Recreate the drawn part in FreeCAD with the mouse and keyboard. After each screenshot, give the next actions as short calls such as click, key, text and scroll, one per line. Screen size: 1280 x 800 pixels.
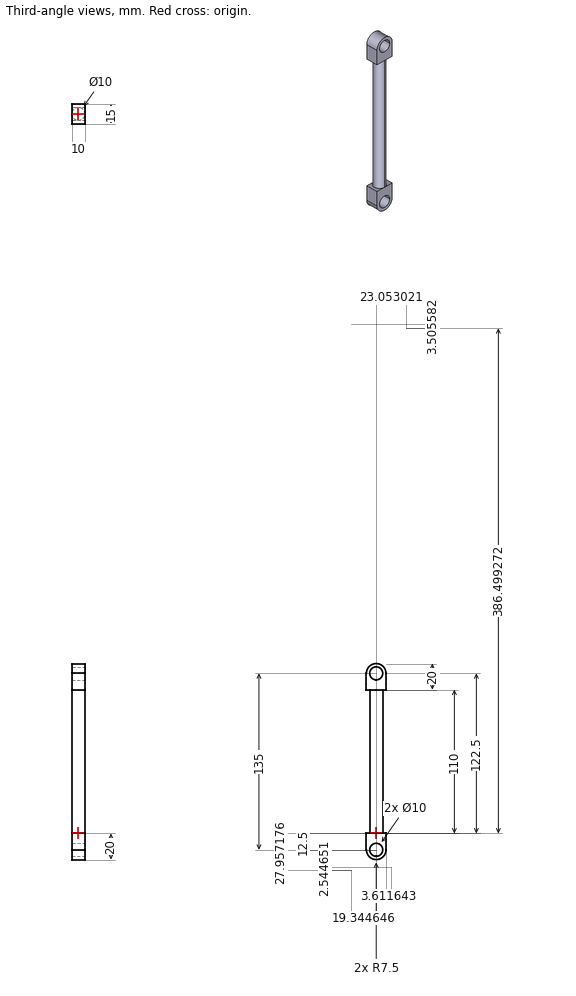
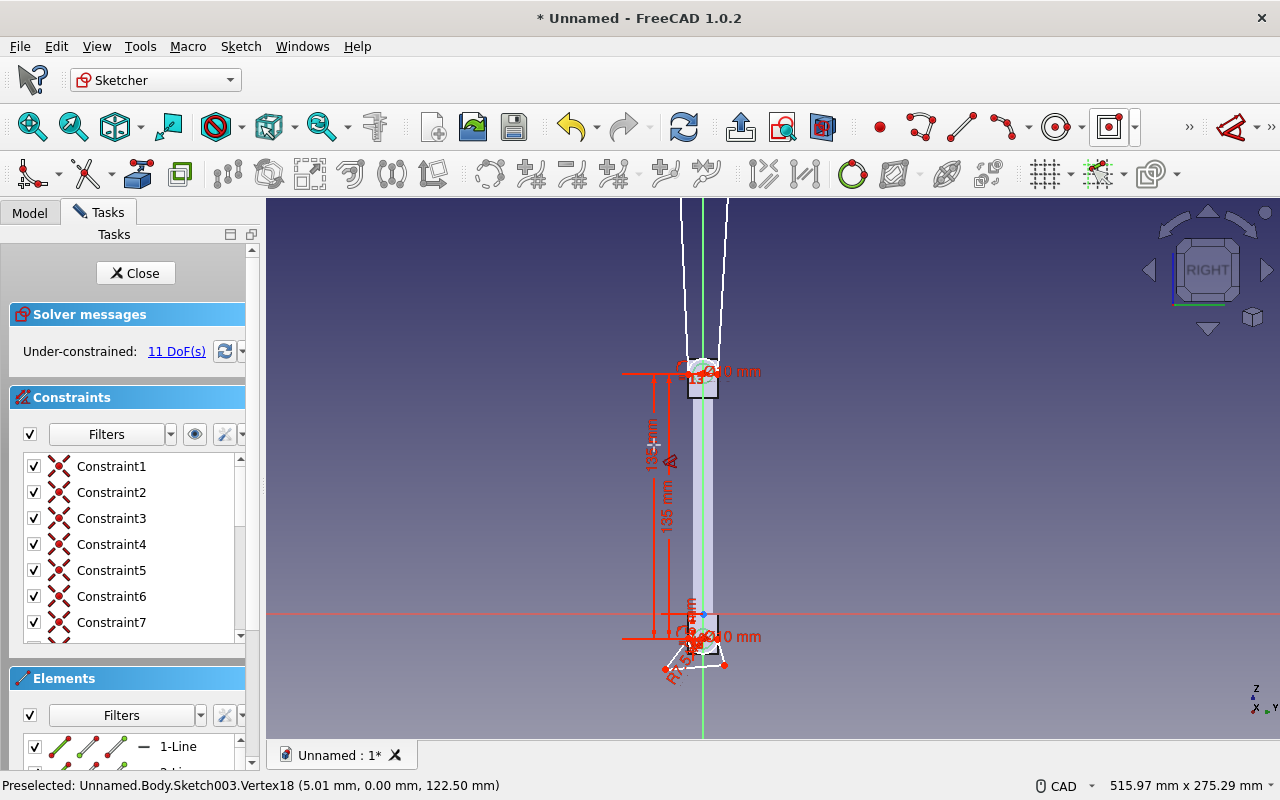
scroll(718, 640, up, 3)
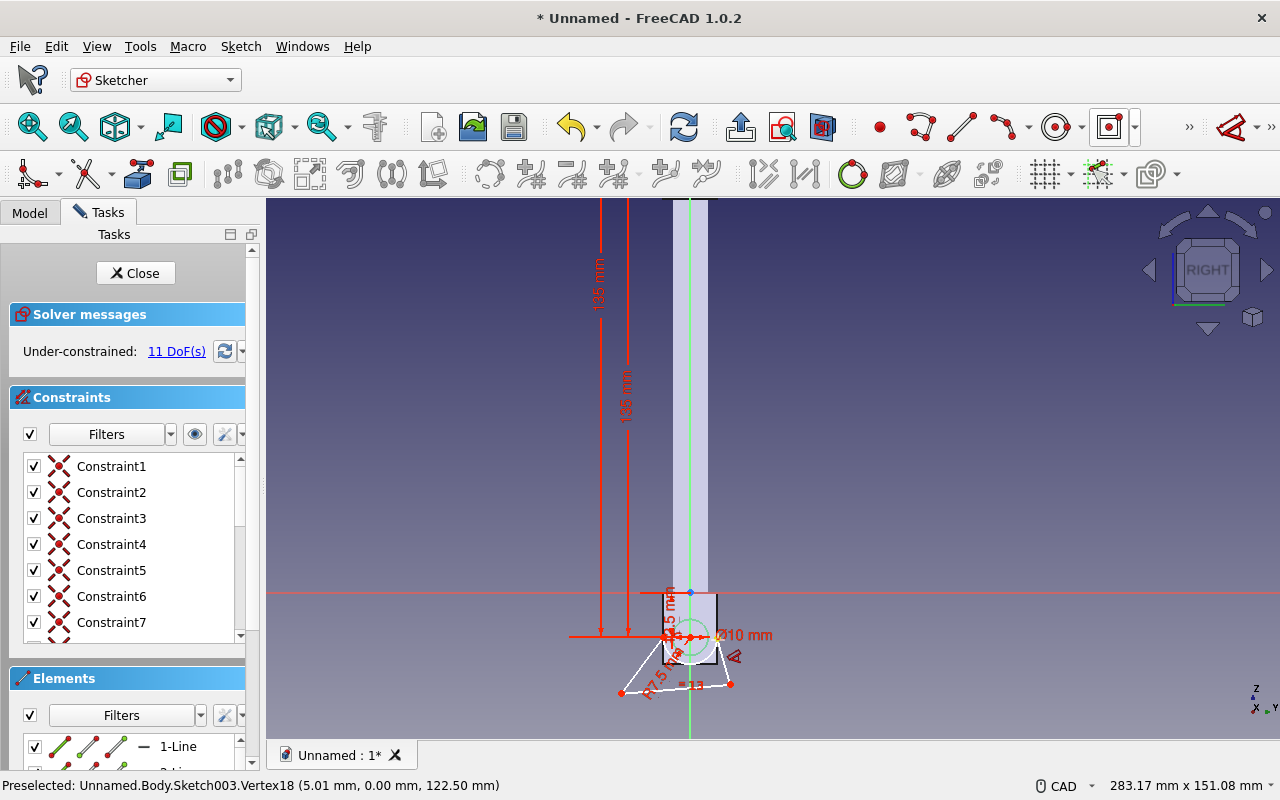
click(717, 639)
click(751, 616)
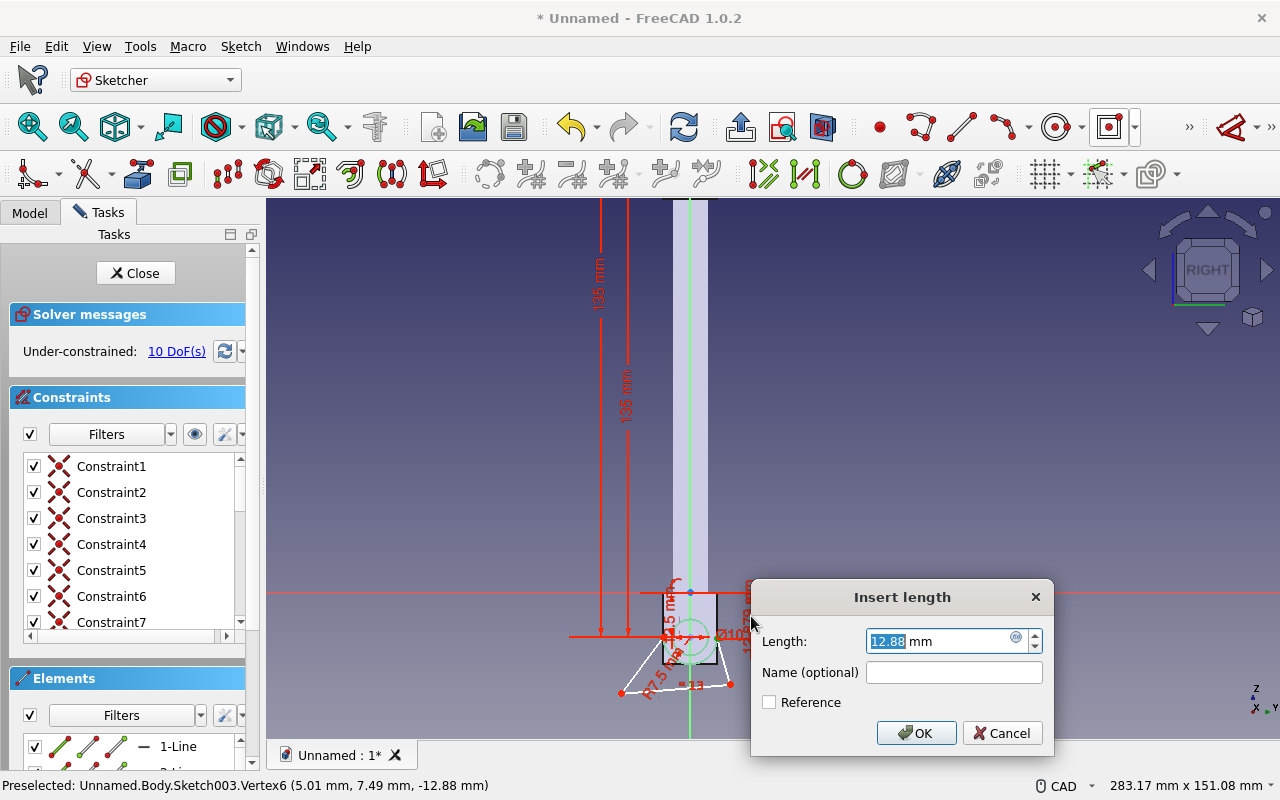
text(12.5)
key(Return)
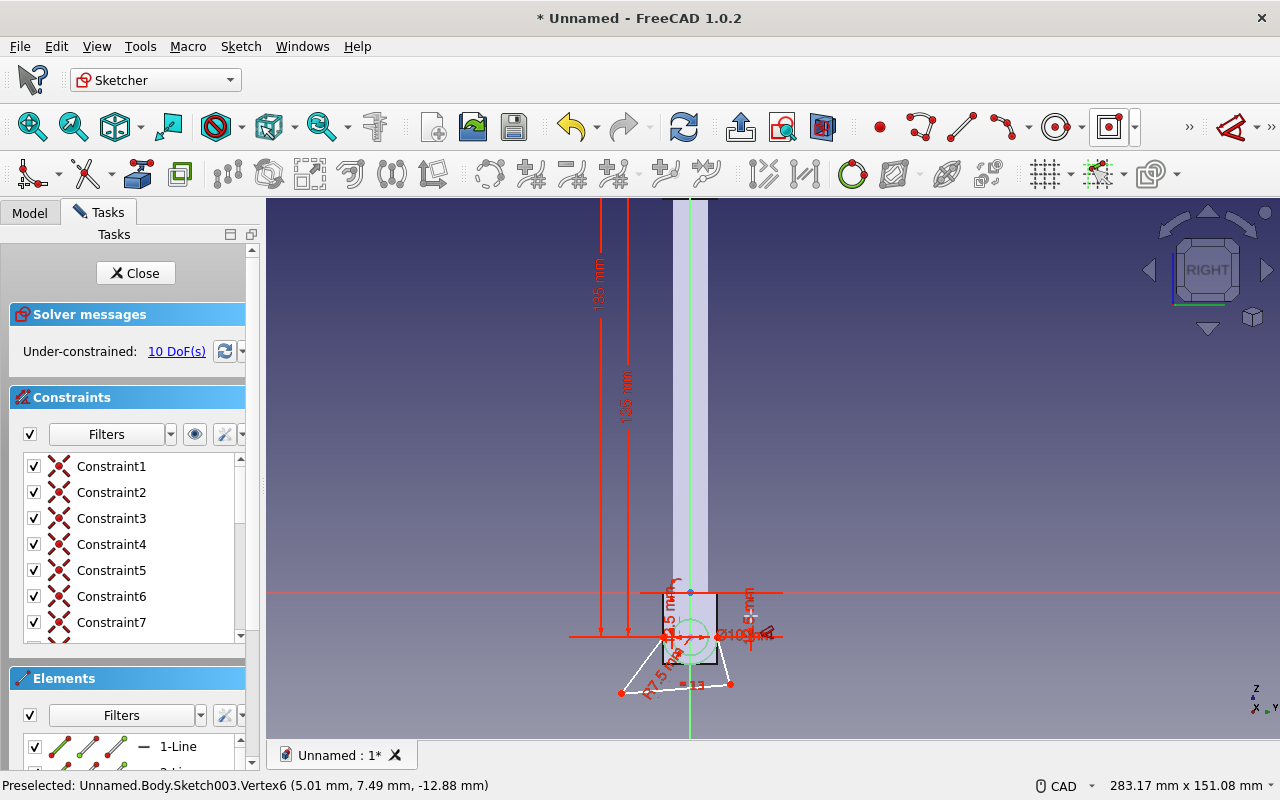
scroll(707, 640, down, 7)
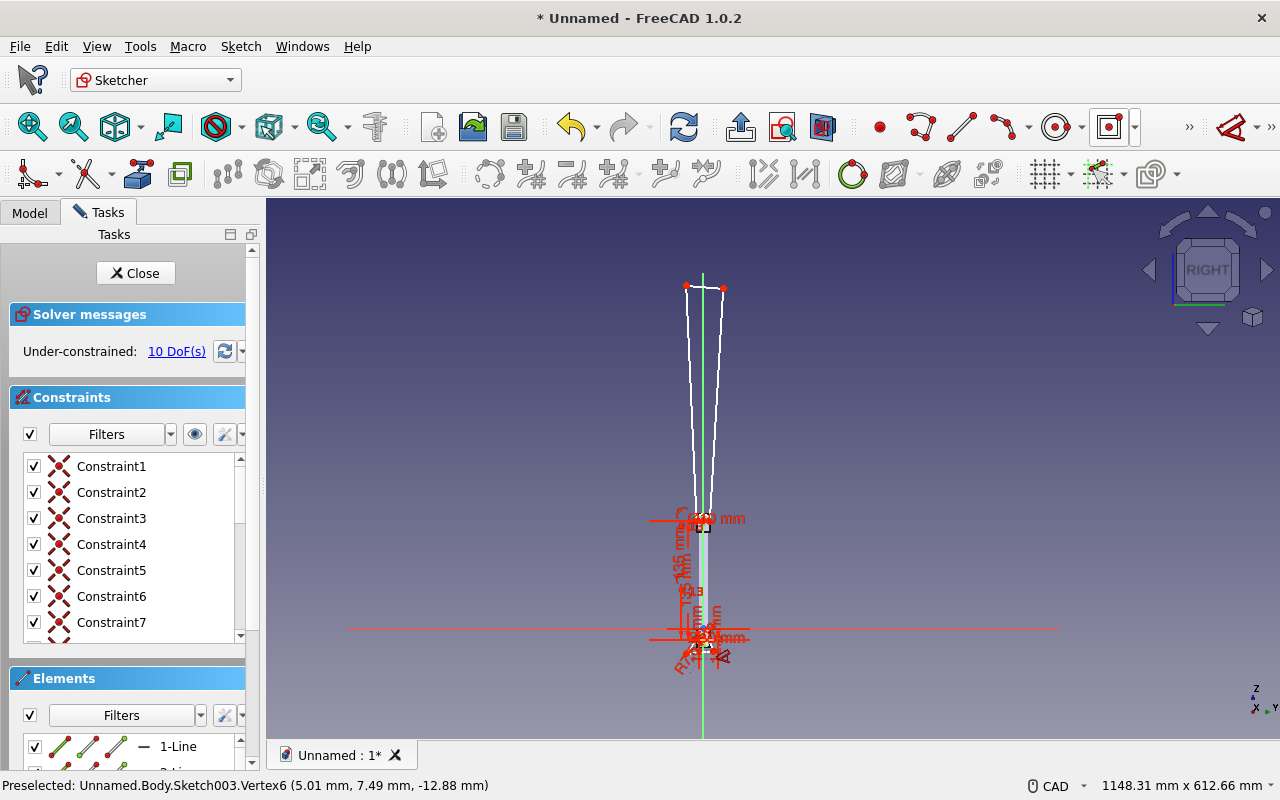
scroll(710, 521, up, 4)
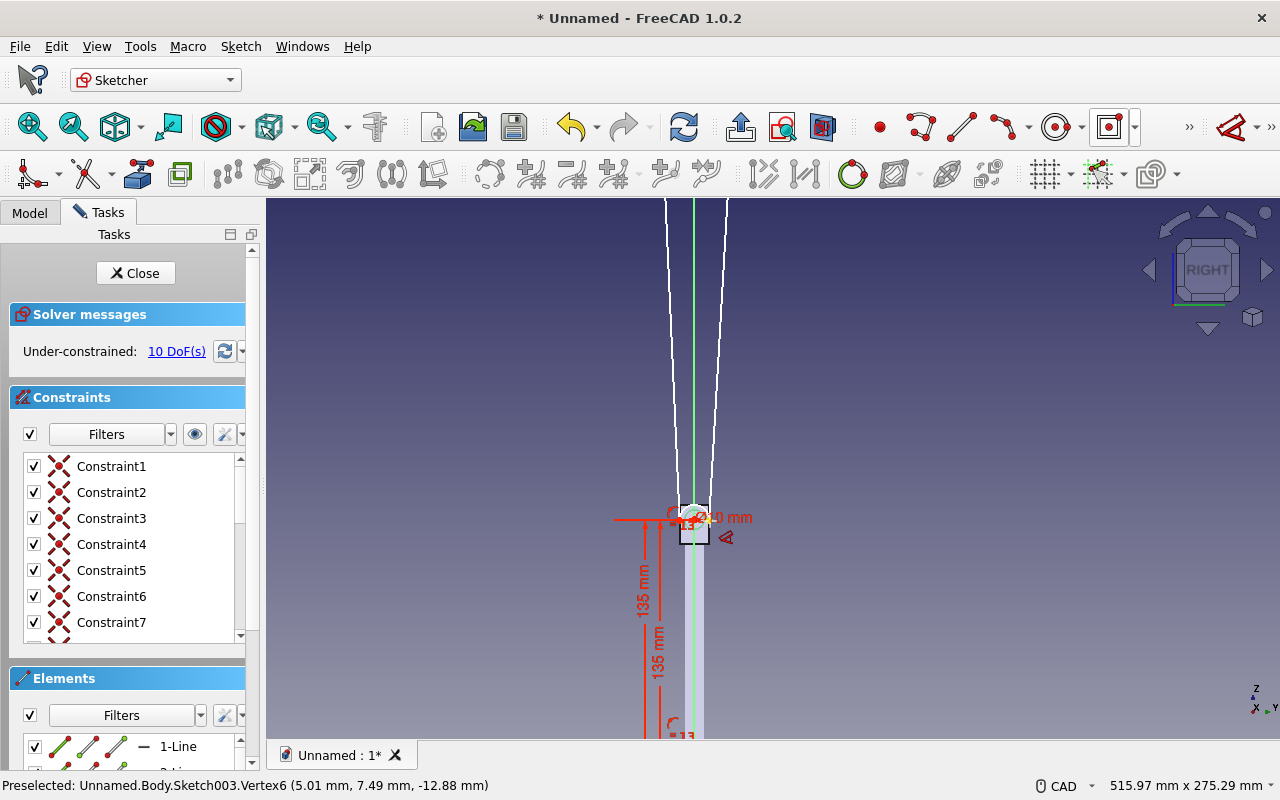
click(709, 521)
click(743, 616)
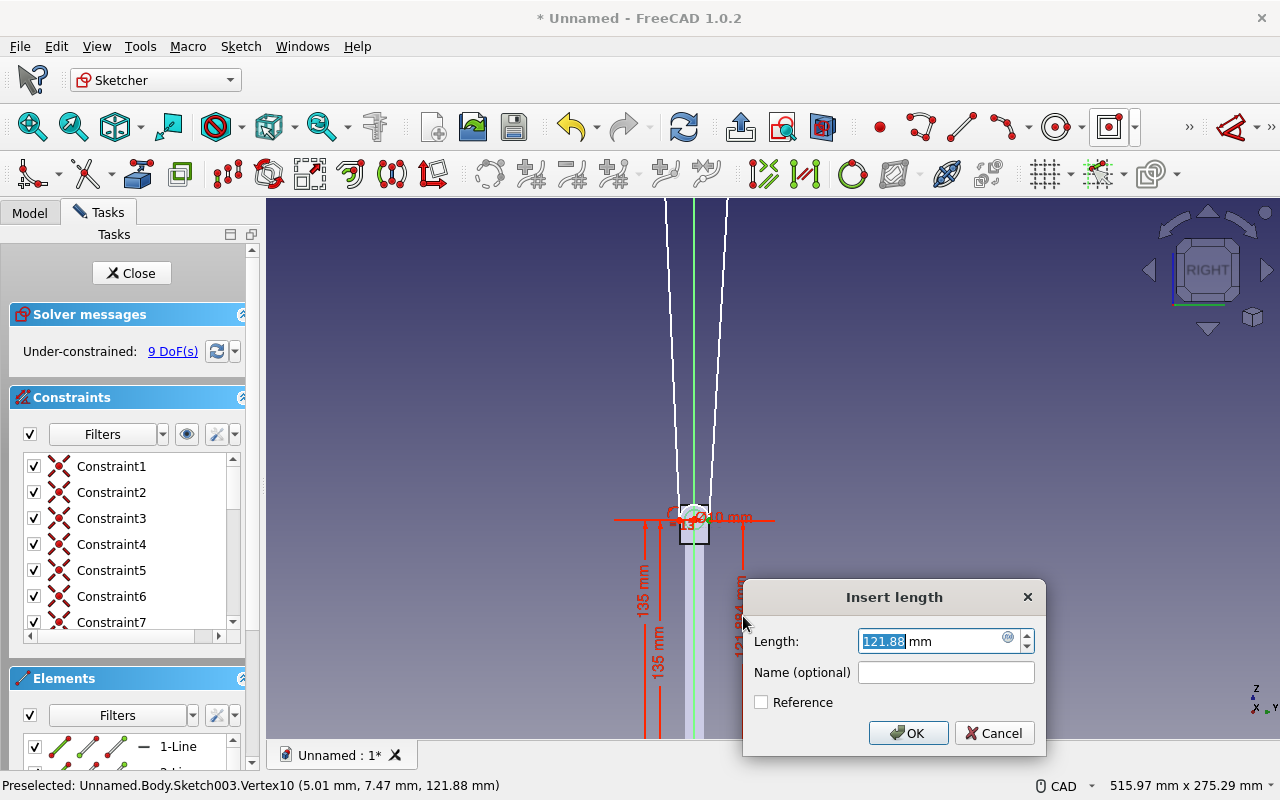
text(122.5)
key(Return)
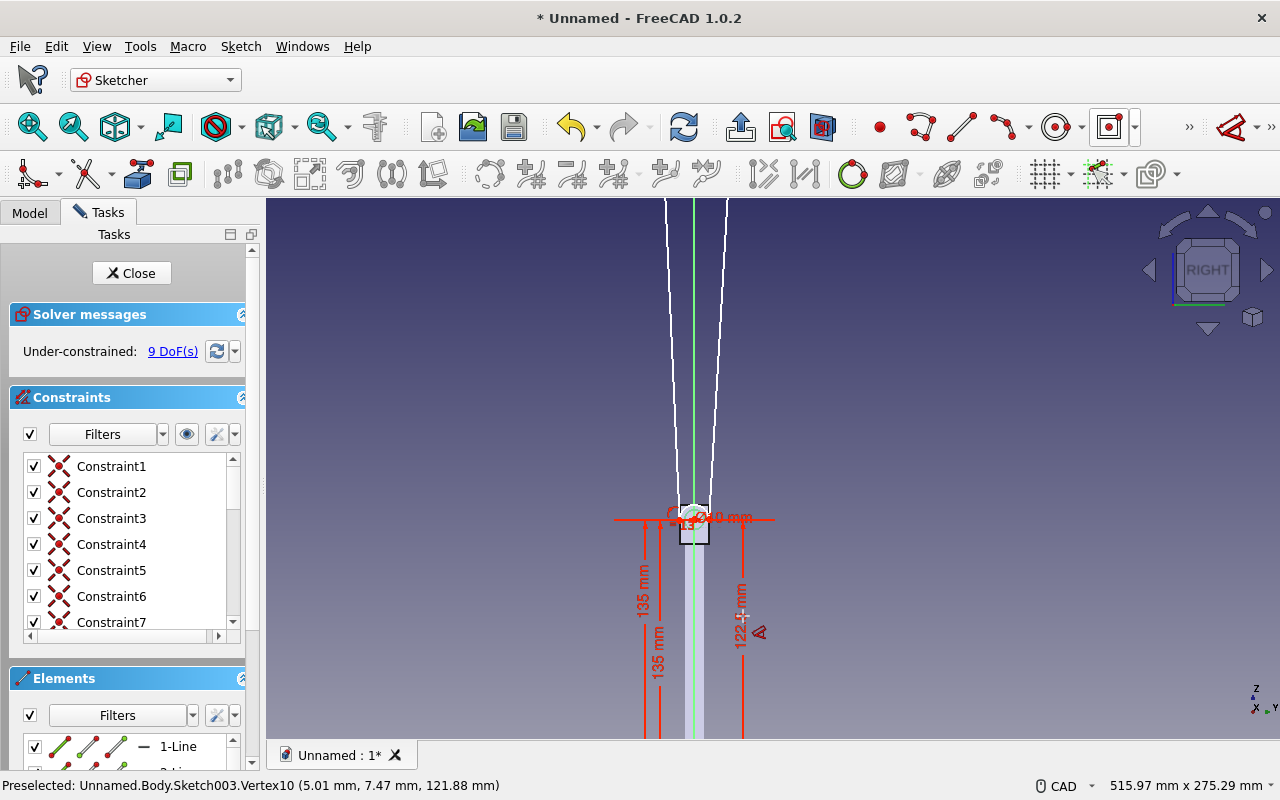
click(680, 521)
click(646, 616)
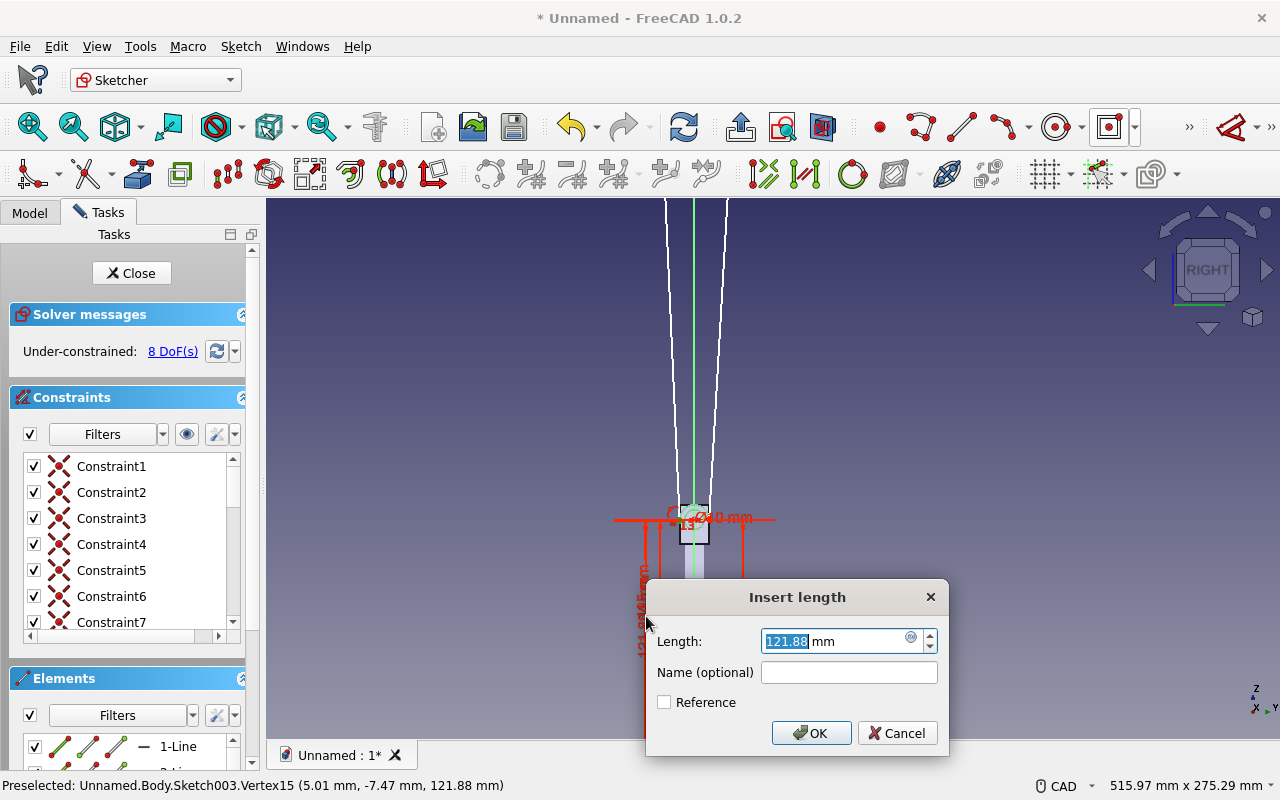
text(122.5)
key(Return)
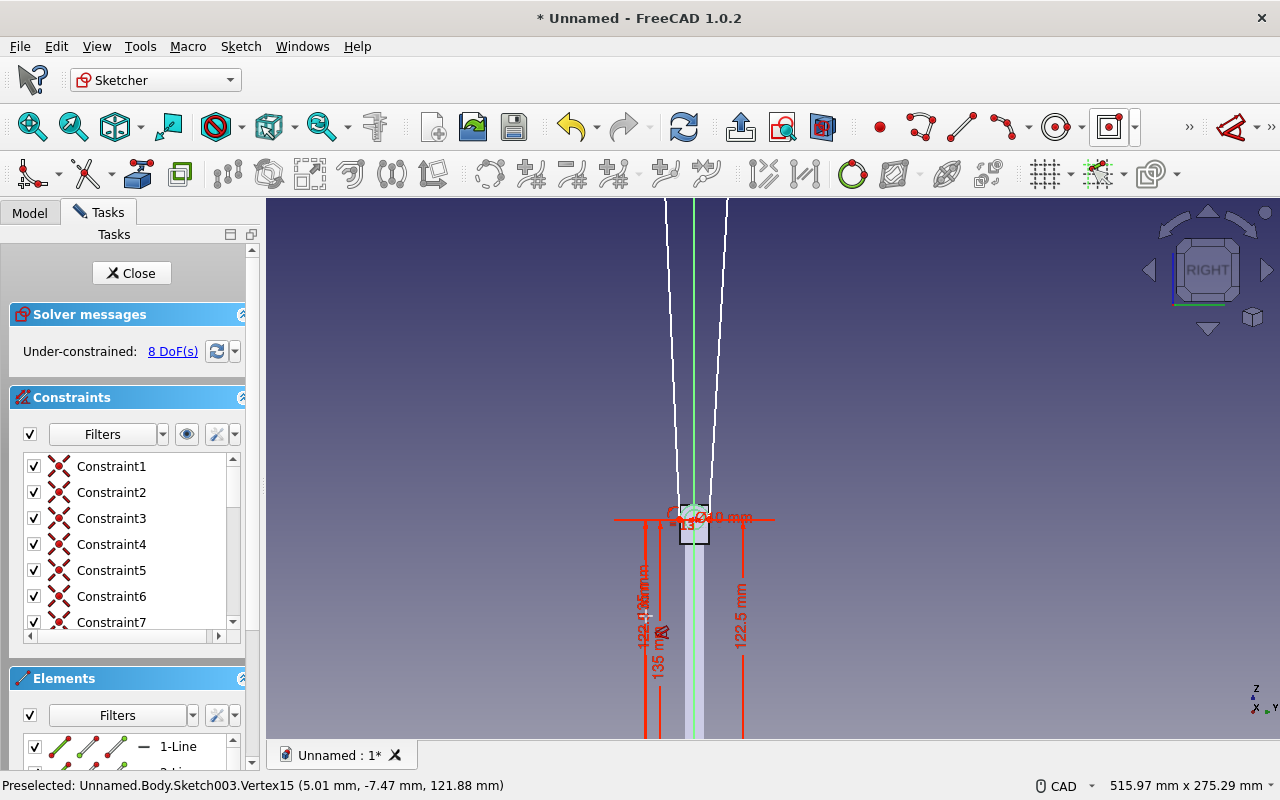
scroll(710, 521, down, 4)